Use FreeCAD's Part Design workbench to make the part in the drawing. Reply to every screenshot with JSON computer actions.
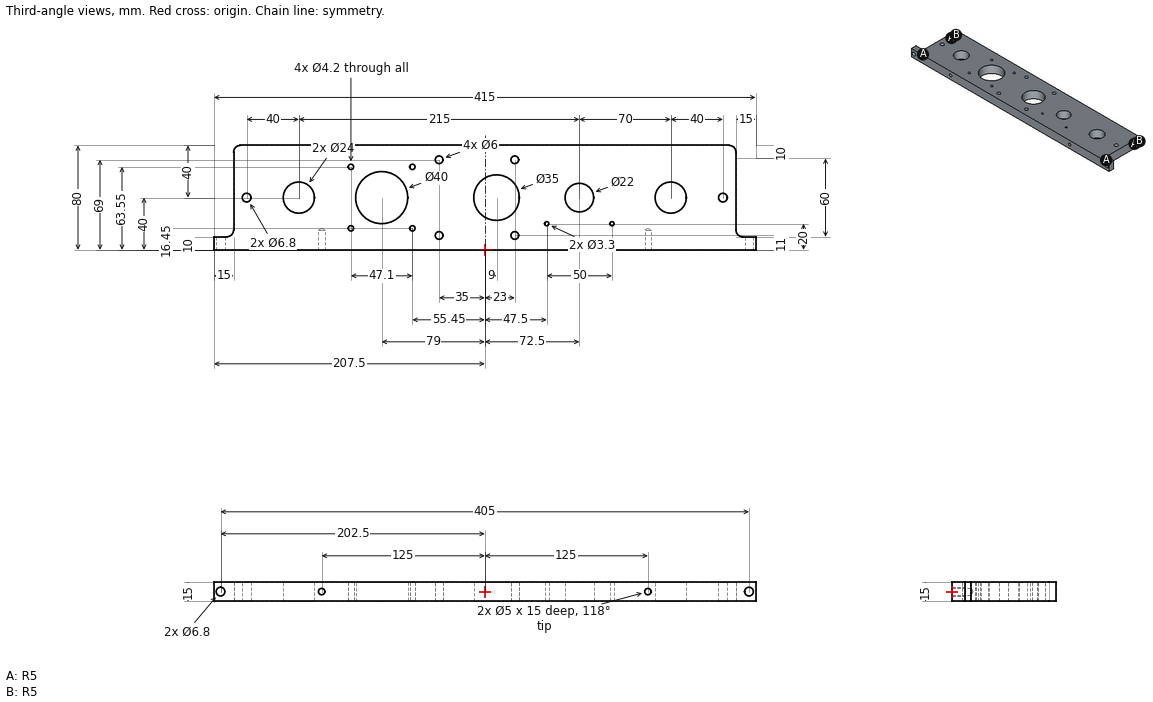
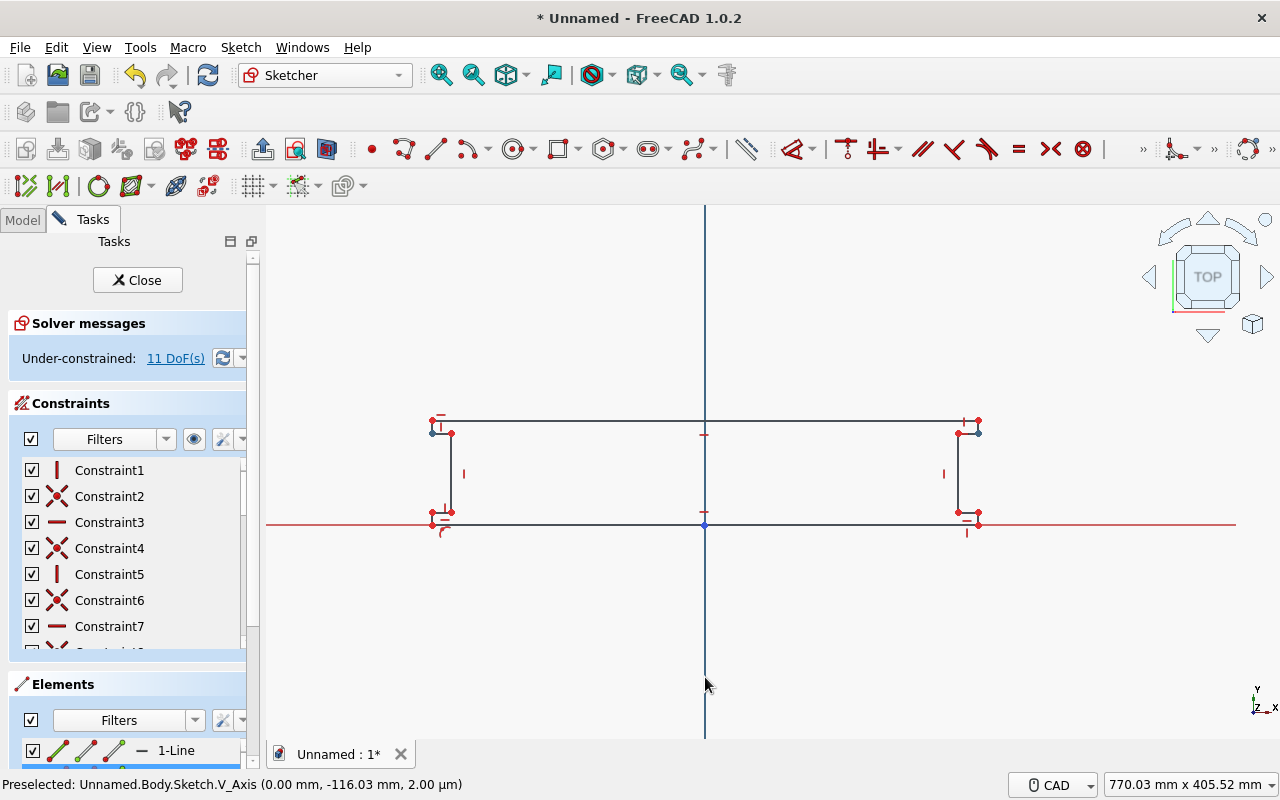
{"action": "left_click", "coordinate": [1052, 150]}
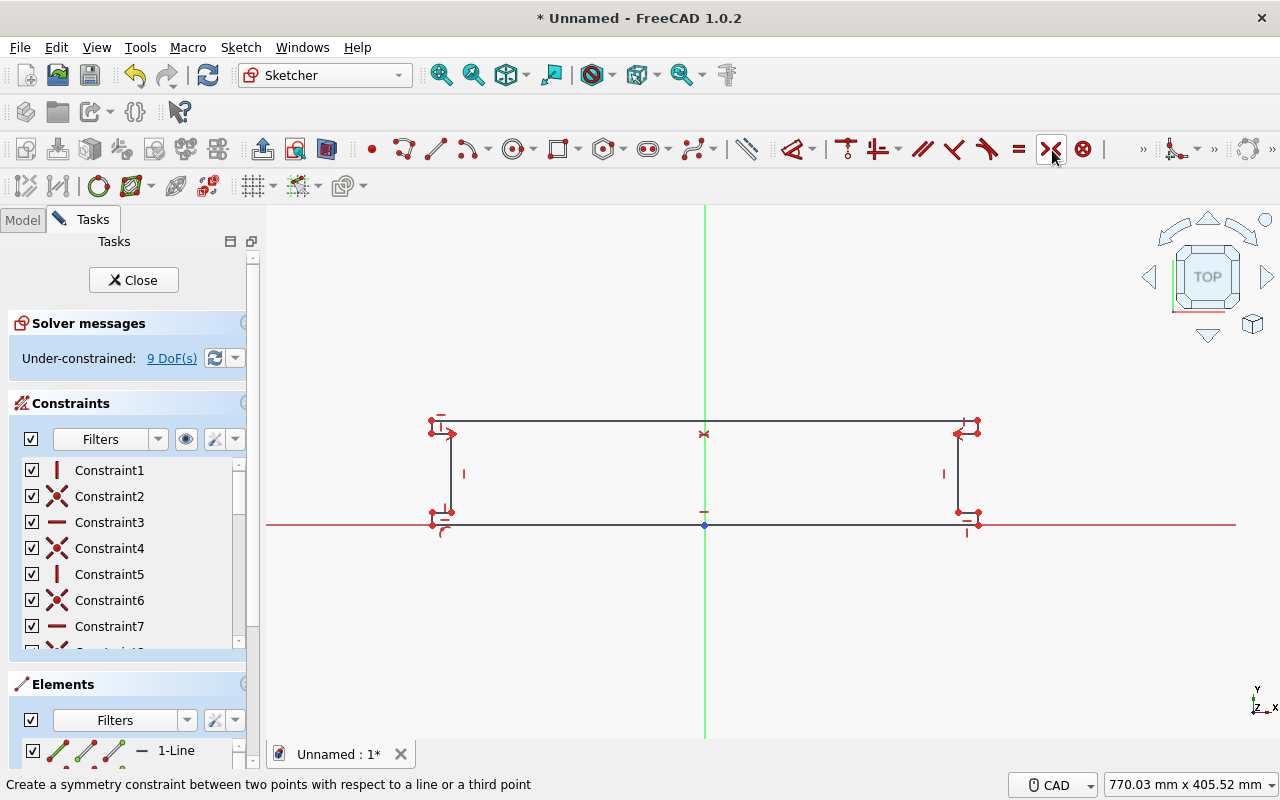
{"action": "left_click", "coordinate": [958, 513]}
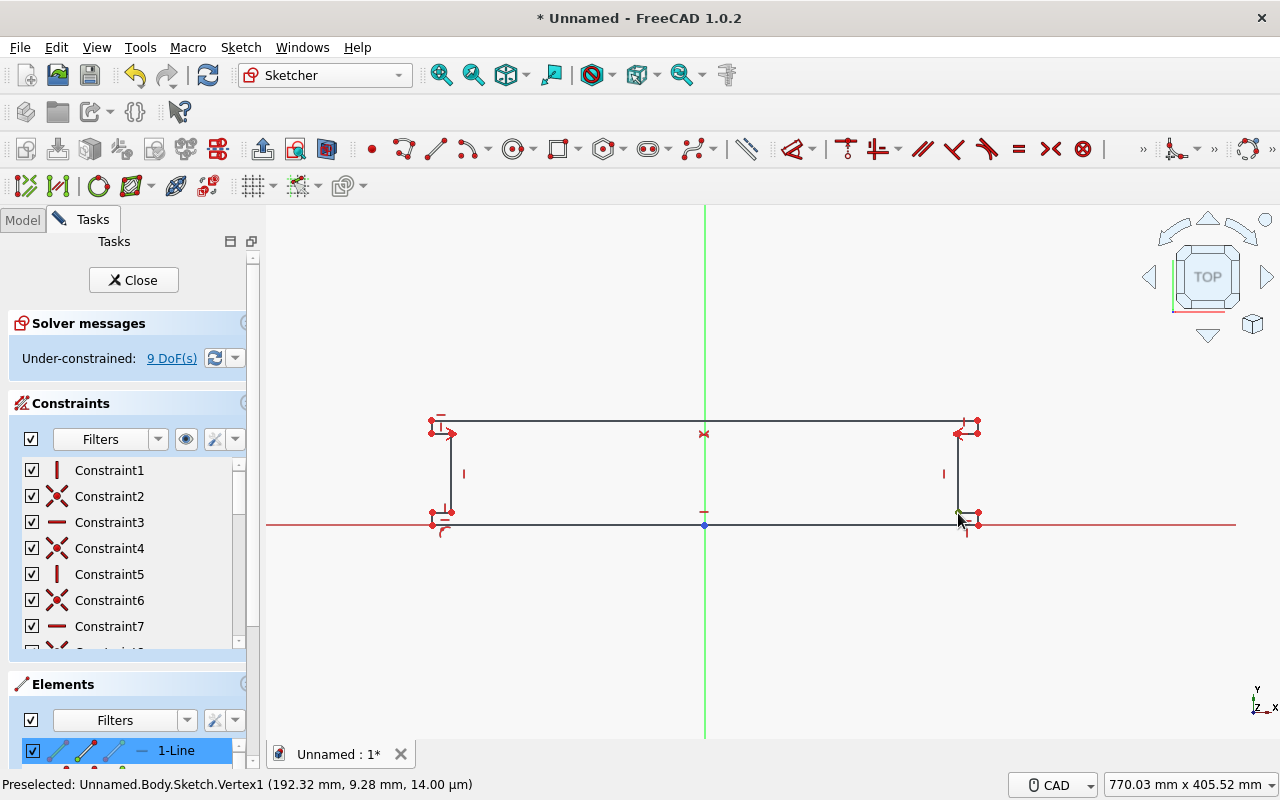
{"action": "left_click", "coordinate": [451, 513]}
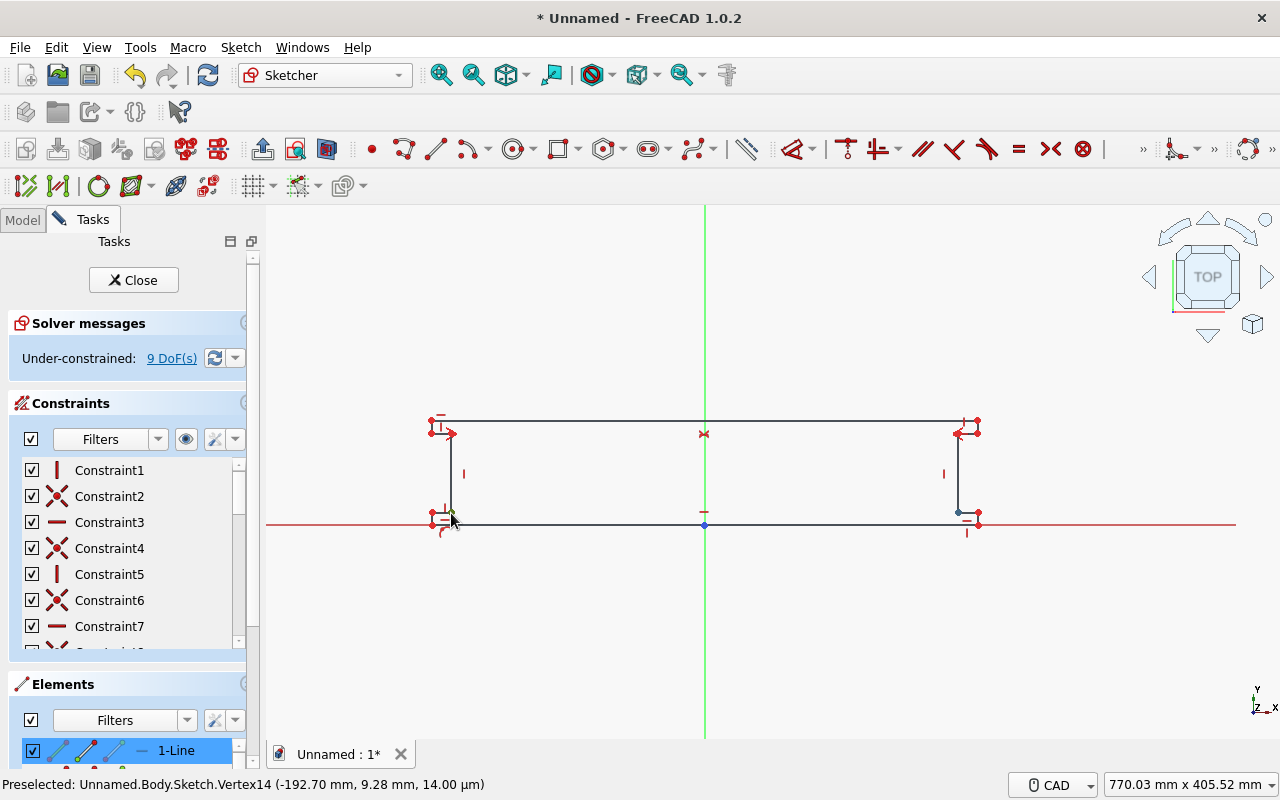
{"action": "left_click", "coordinate": [705, 677]}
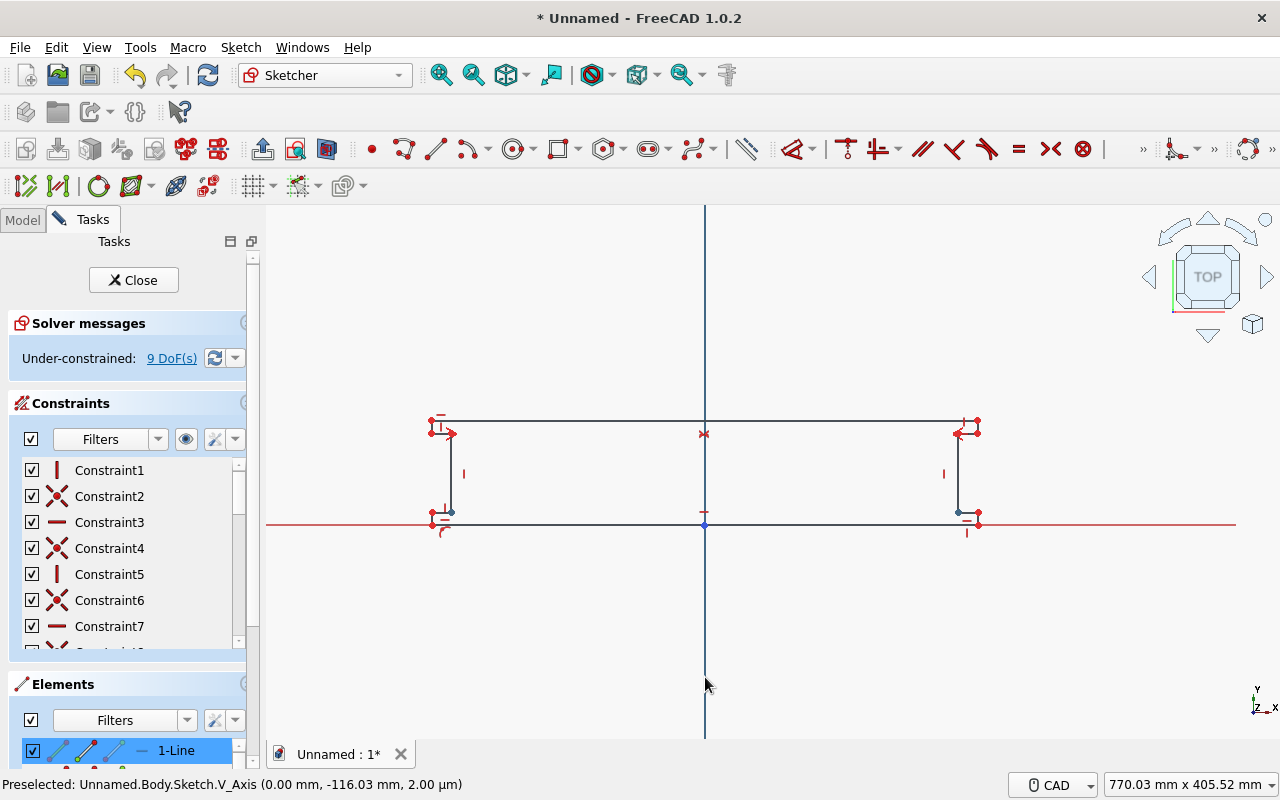
{"action": "left_click", "coordinate": [1052, 150]}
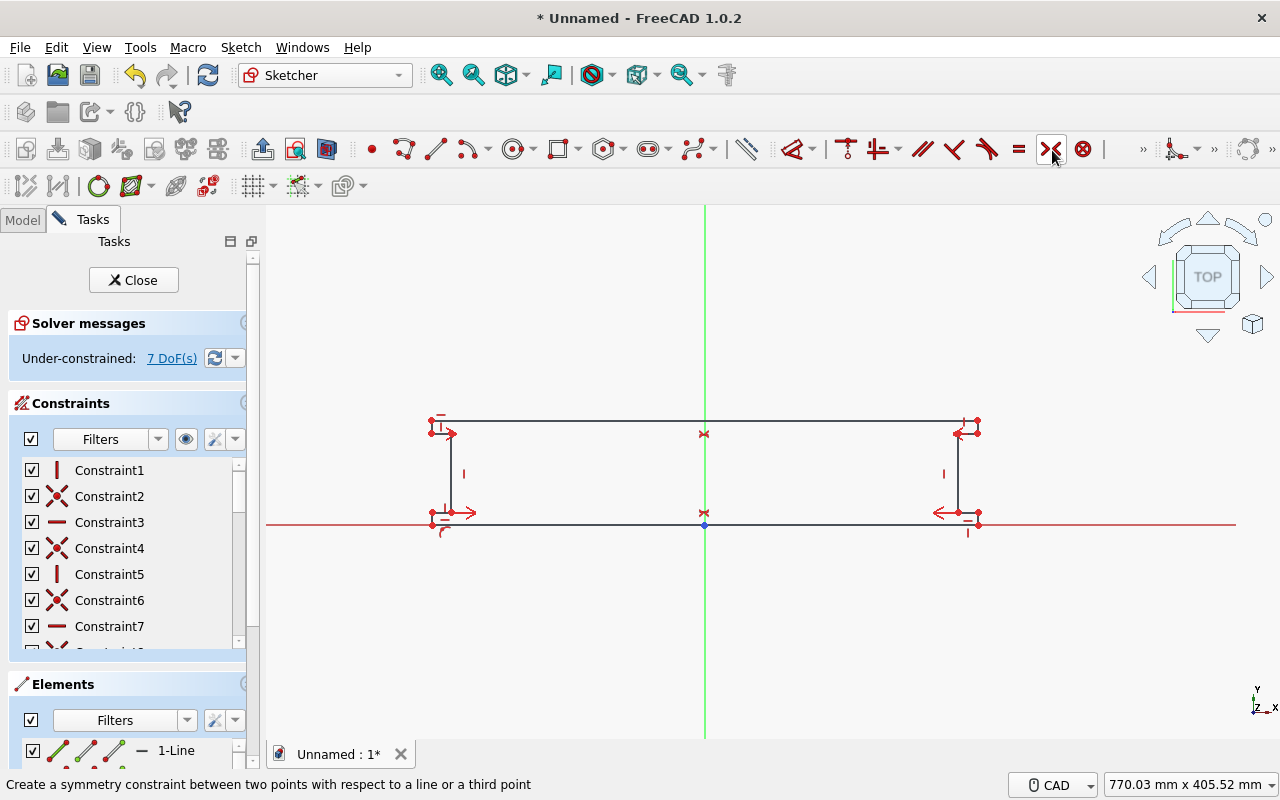
{"action": "left_click", "coordinate": [792, 150]}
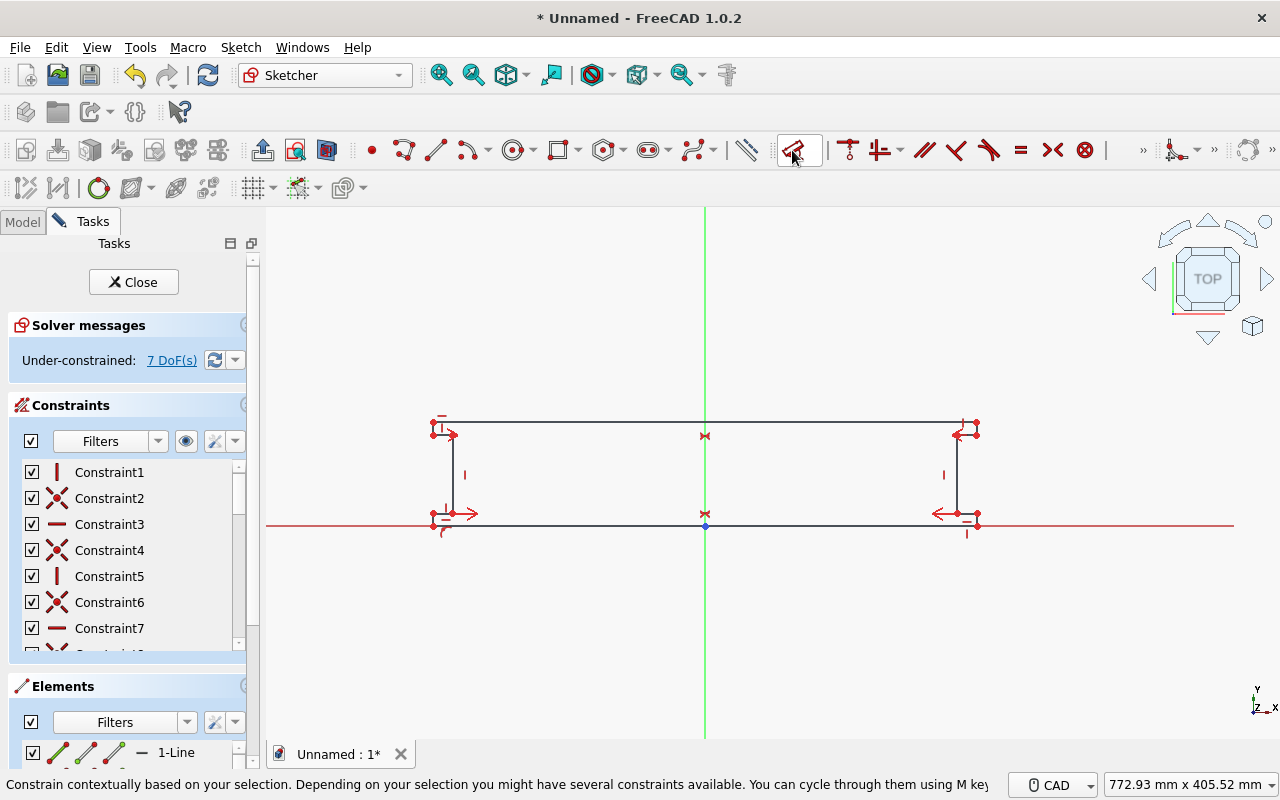
{"action": "left_click", "coordinate": [957, 490]}
{"action": "left_click", "coordinate": [991, 474]}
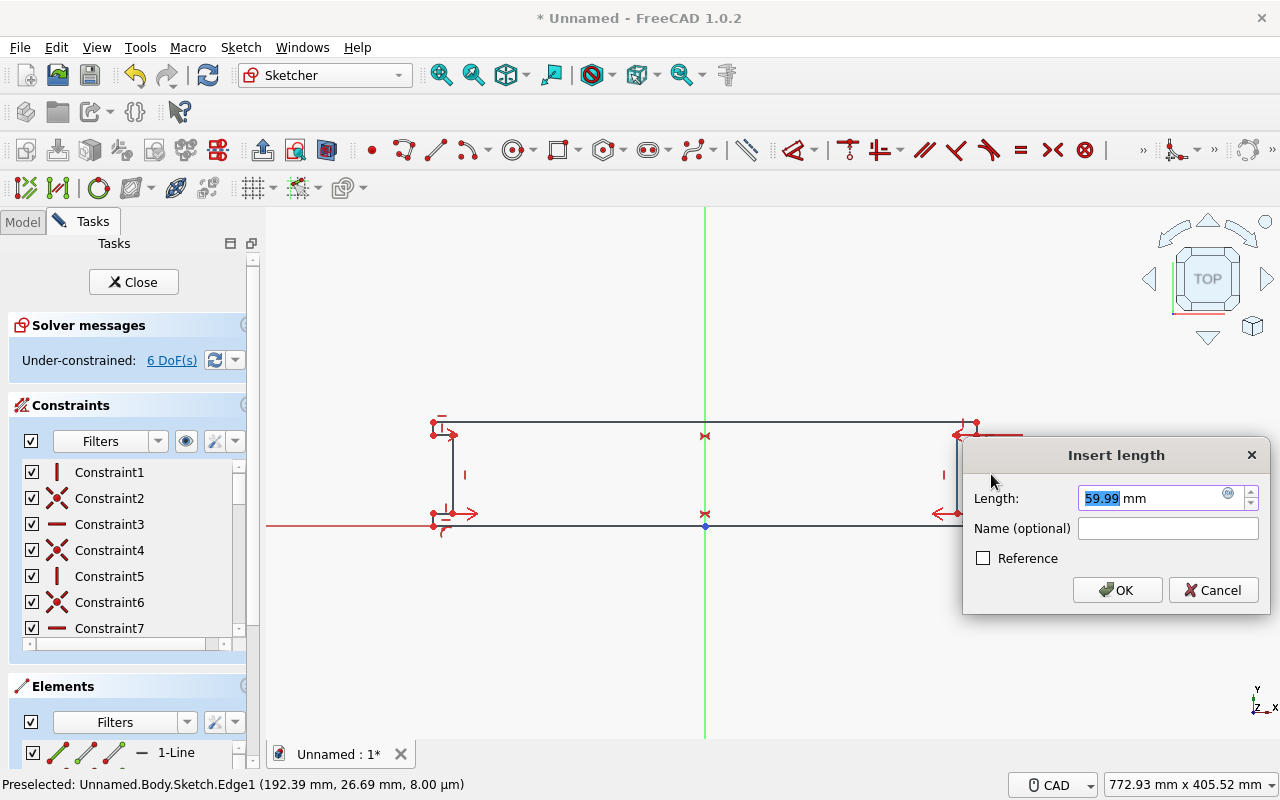
{"action": "type", "text": "60"}
{"action": "key", "text": "Return"}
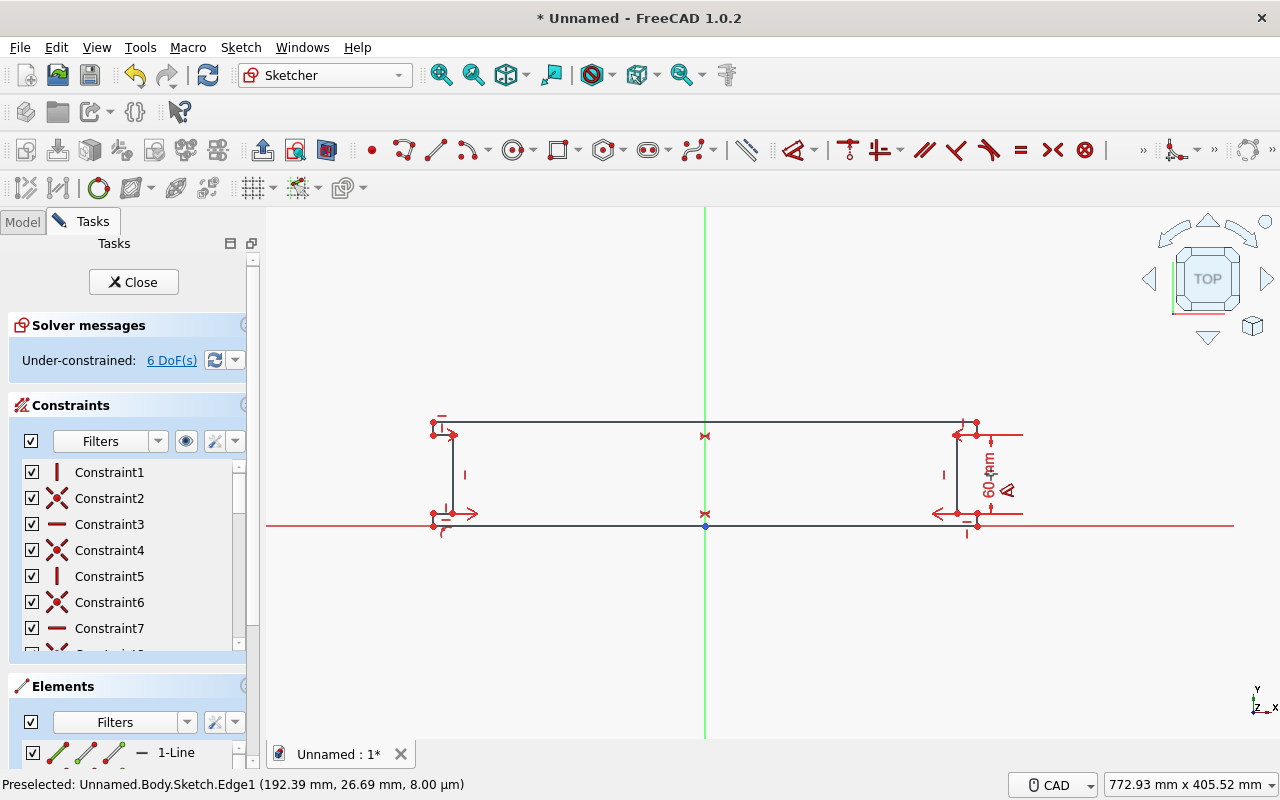
{"action": "scroll", "coordinate": [967, 435], "scroll_direction": "up", "scroll_amount": 4}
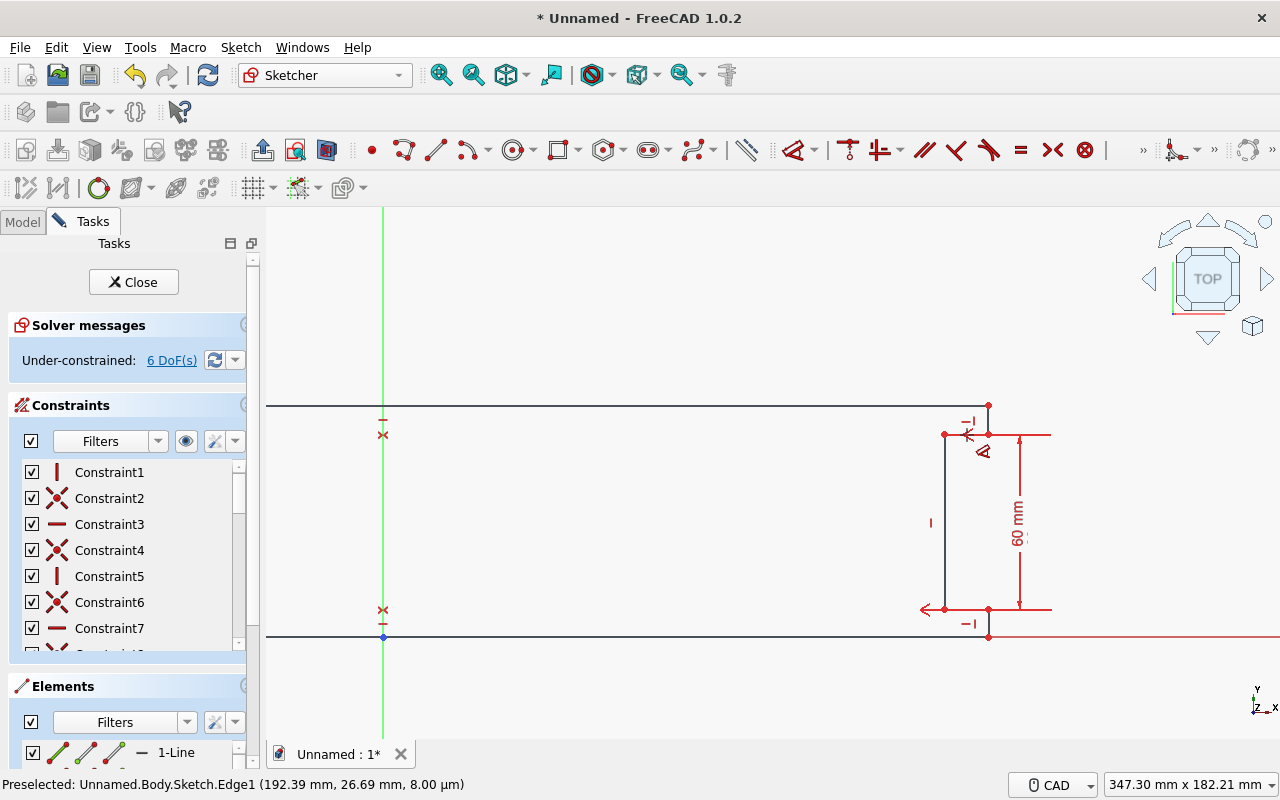
{"action": "left_click", "coordinate": [966, 435]}
{"action": "left_click", "coordinate": [966, 469]}